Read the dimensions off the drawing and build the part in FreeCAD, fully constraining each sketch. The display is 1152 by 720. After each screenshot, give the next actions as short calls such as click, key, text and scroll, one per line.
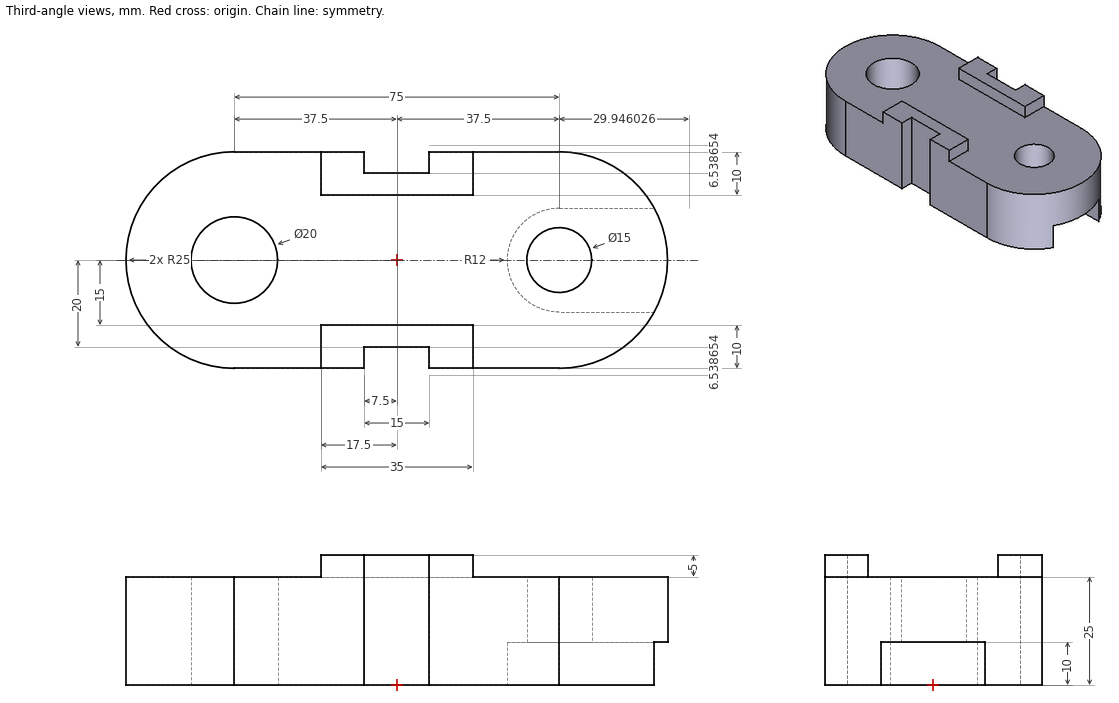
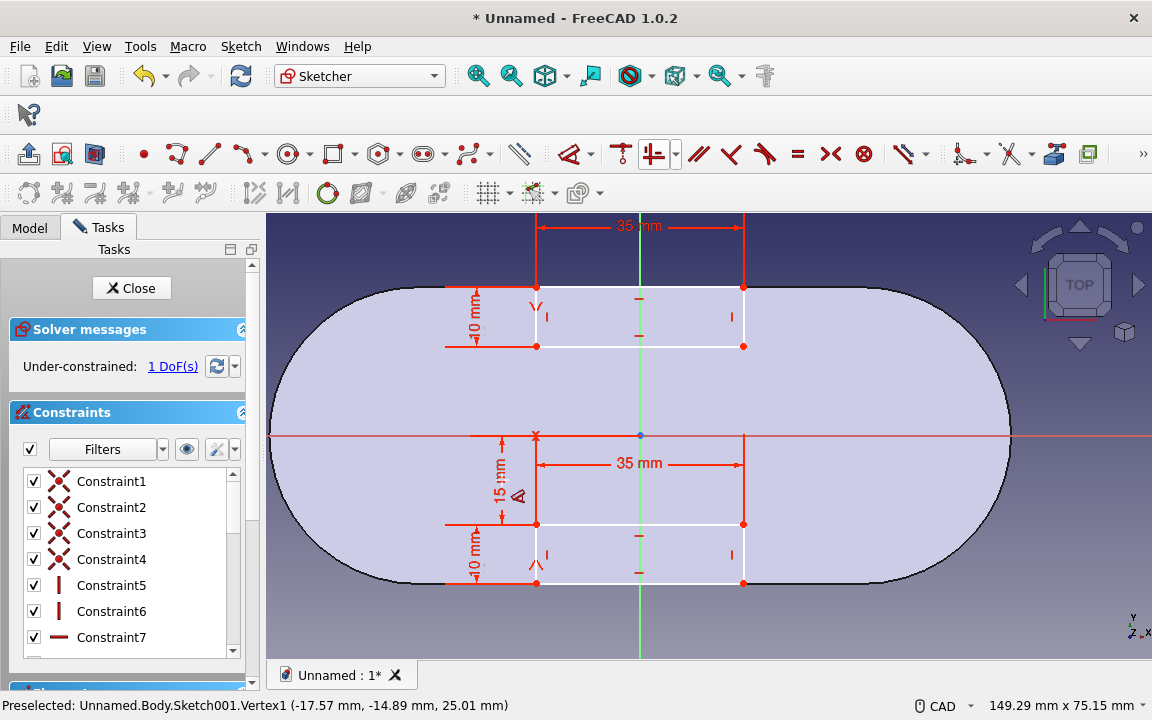
click(536, 525)
click(588, 559)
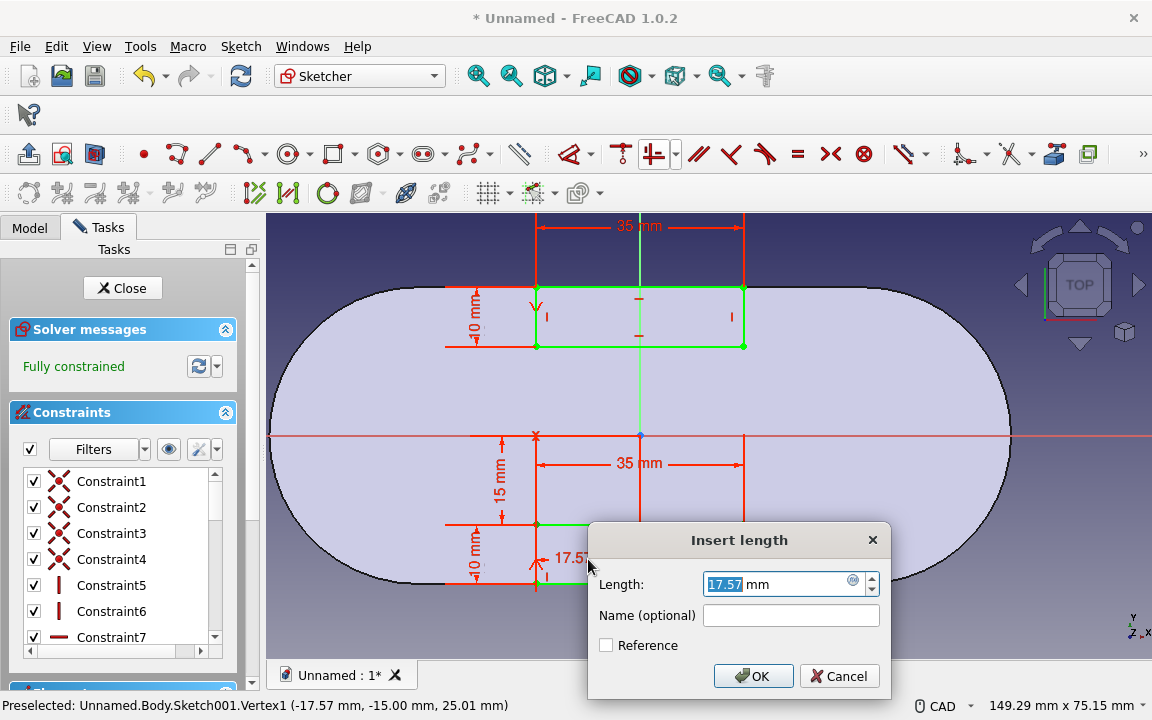
text(17.5)
key(Return)
key(Escape)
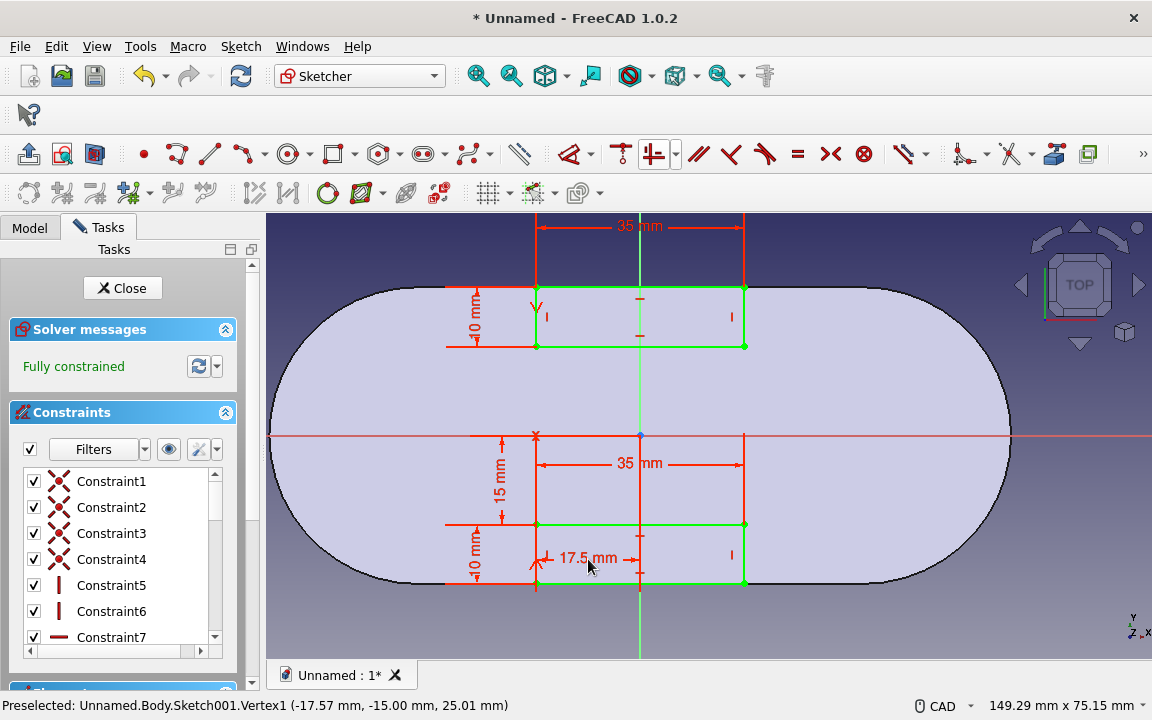
click(123, 288)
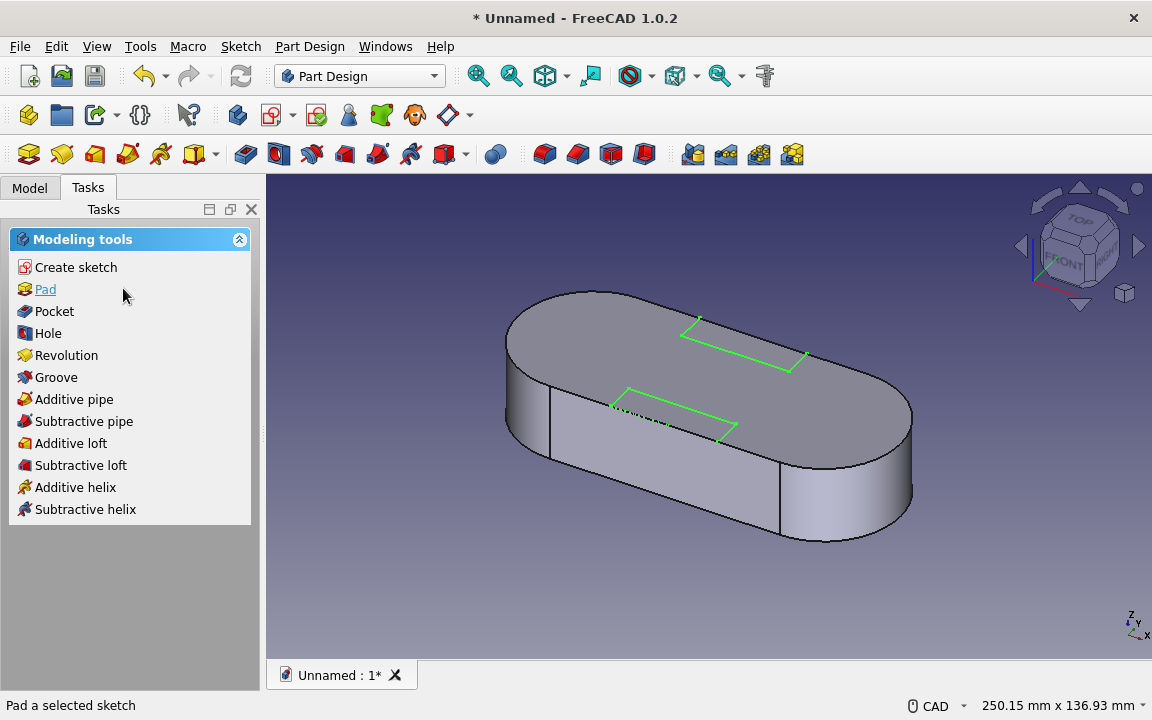
click(29, 154)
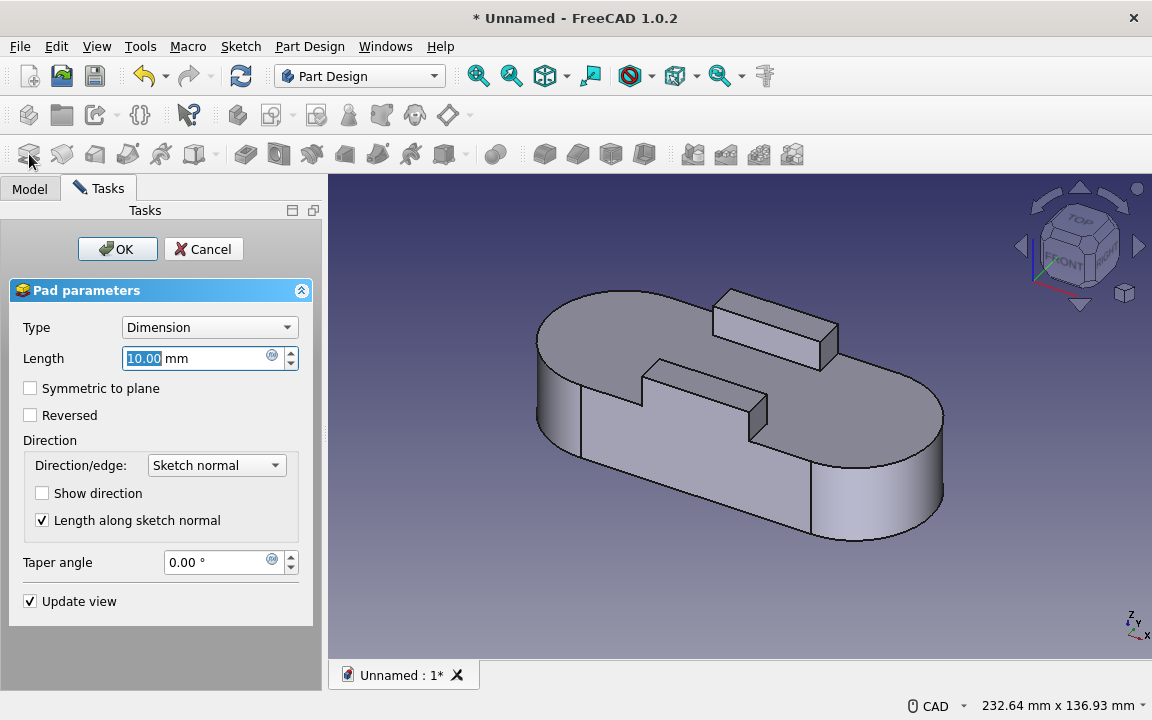
text(5)
key(Tab)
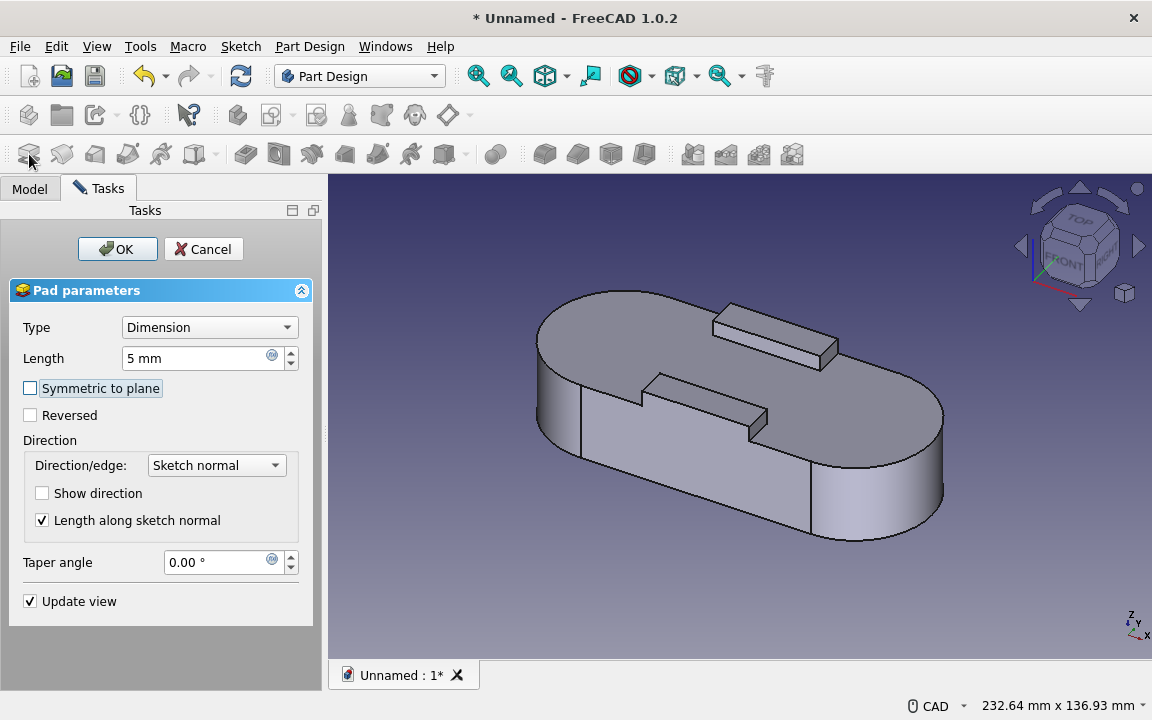
click(118, 249)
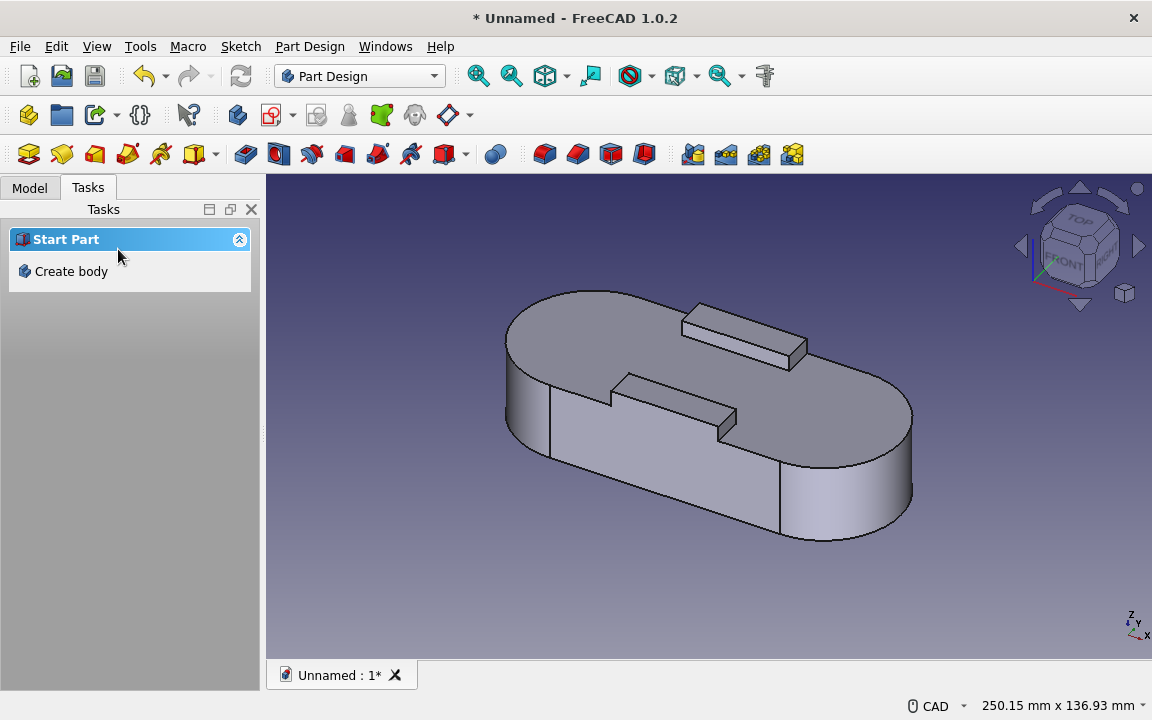
click(704, 409)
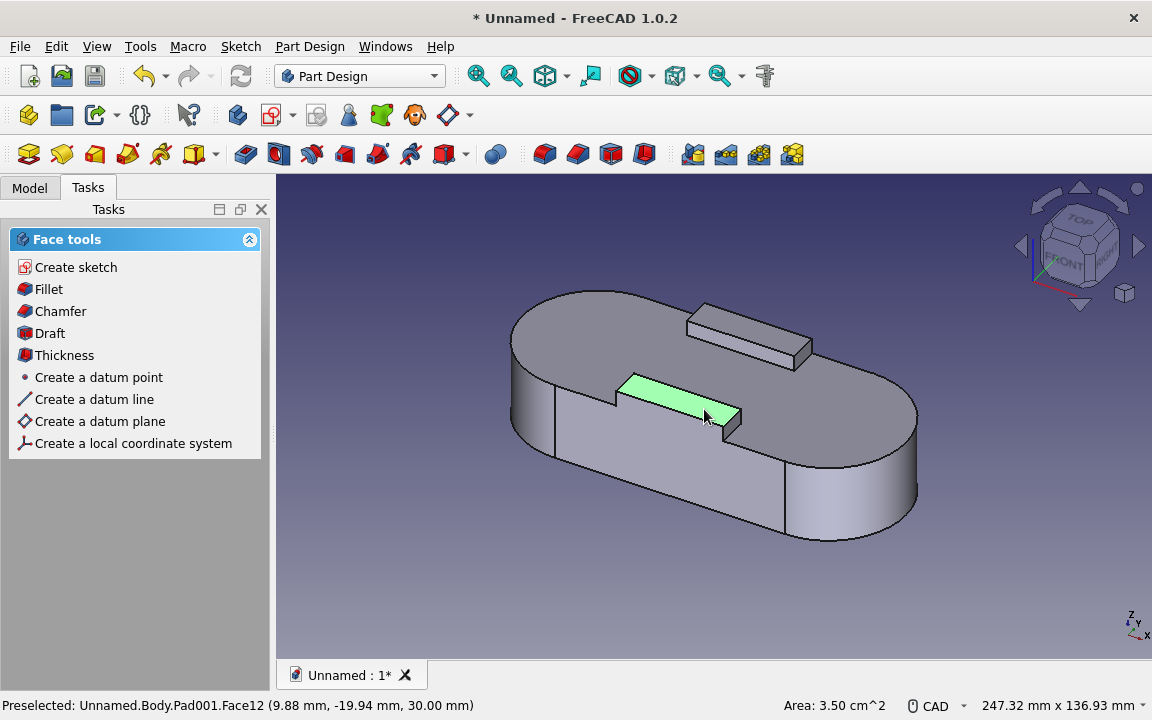
click(270, 116)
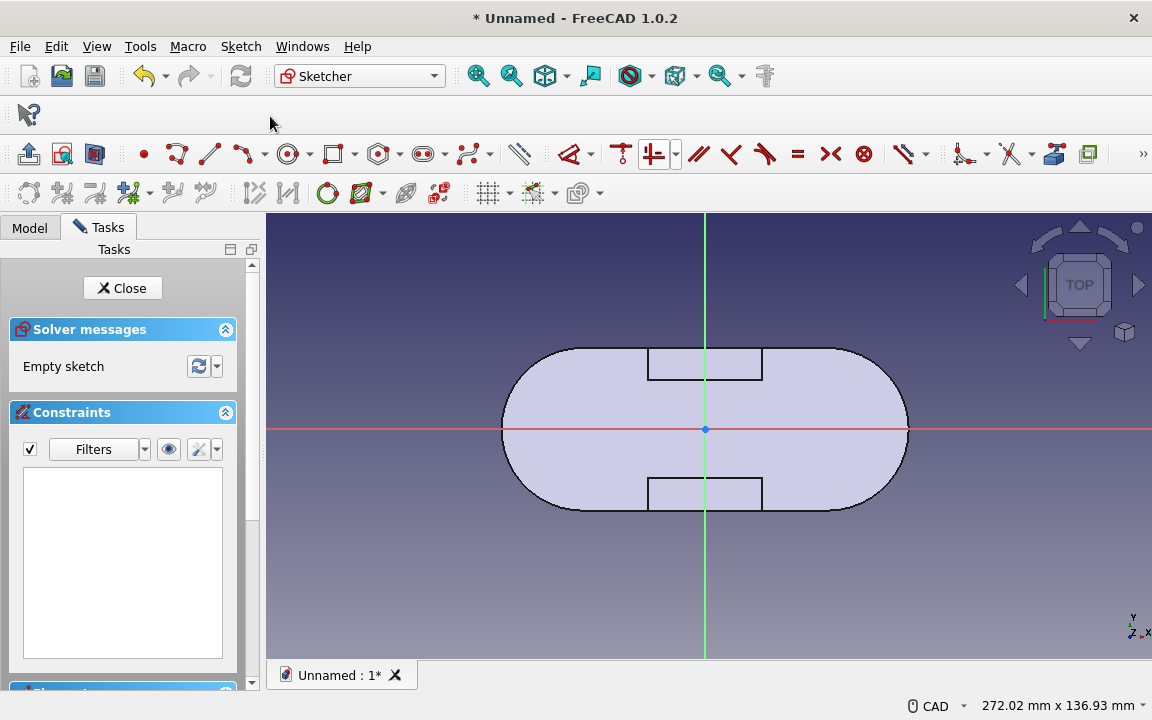
scroll(837, 416, up, 2)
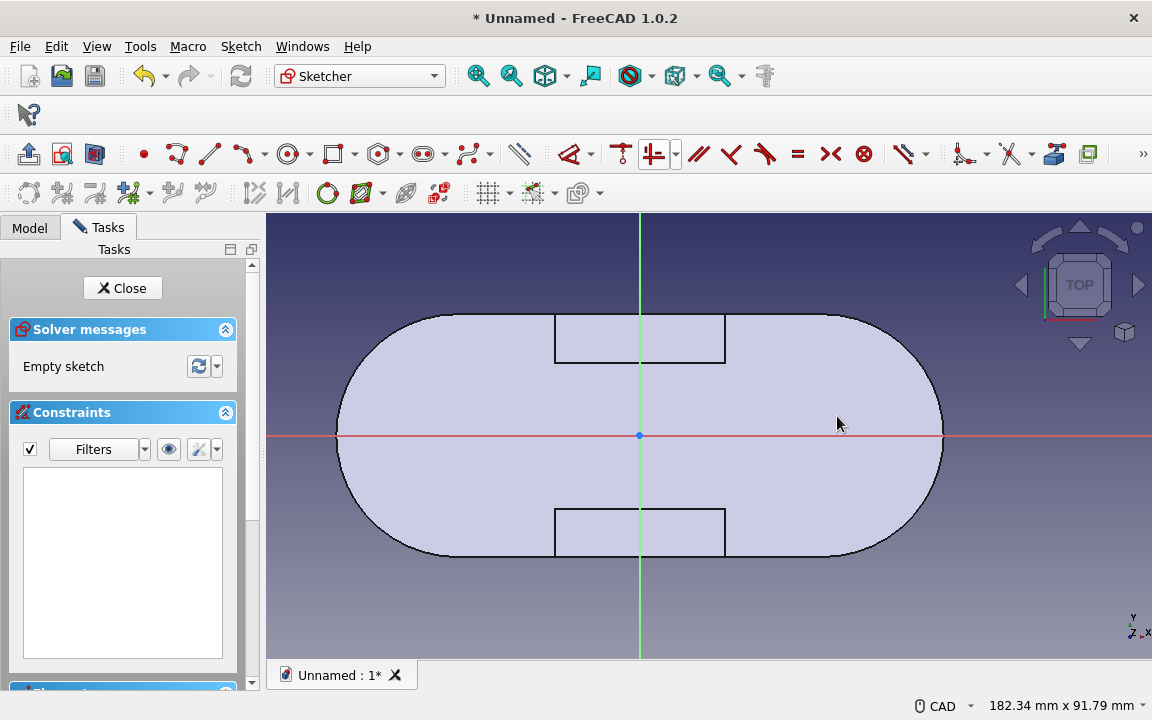
click(332, 154)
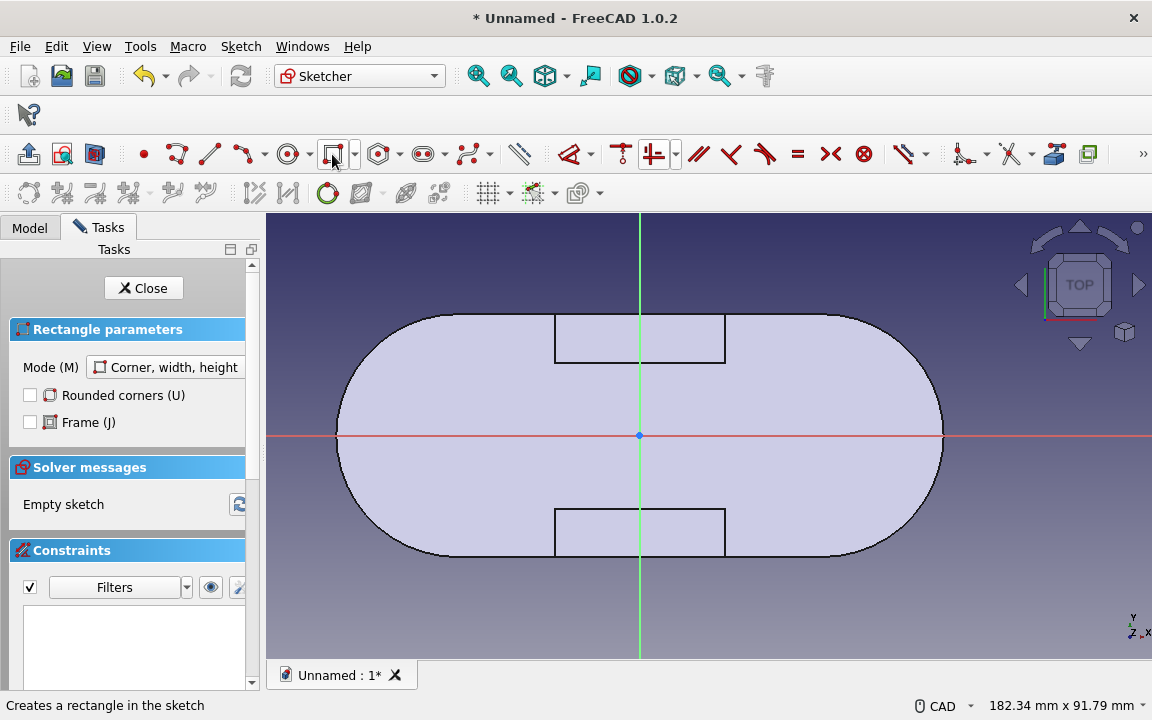
click(604, 533)
move(676, 565)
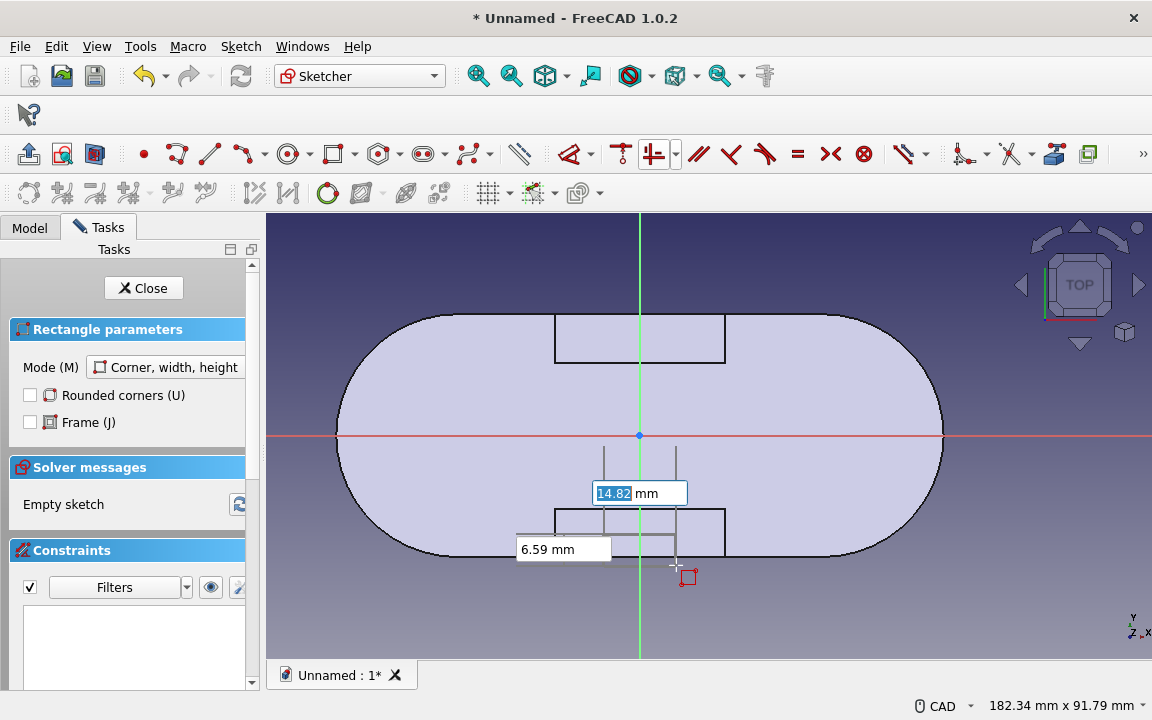
text(15)
key(Tab)
text(6.538654)
key(Return)